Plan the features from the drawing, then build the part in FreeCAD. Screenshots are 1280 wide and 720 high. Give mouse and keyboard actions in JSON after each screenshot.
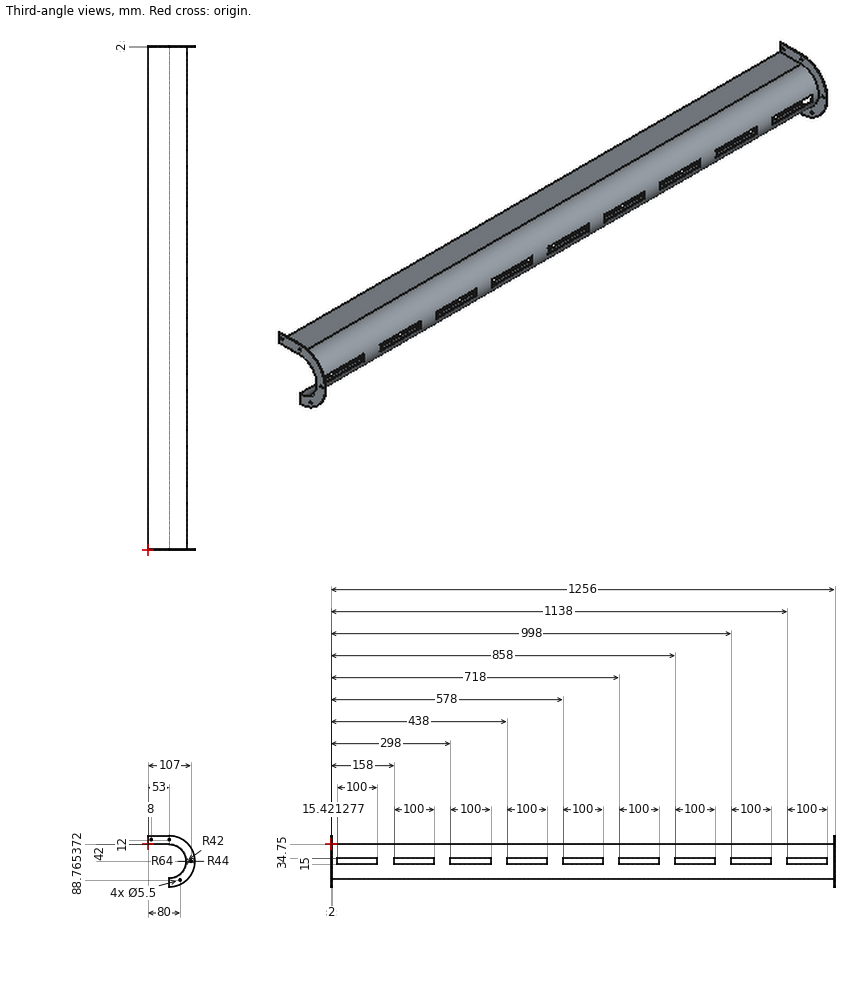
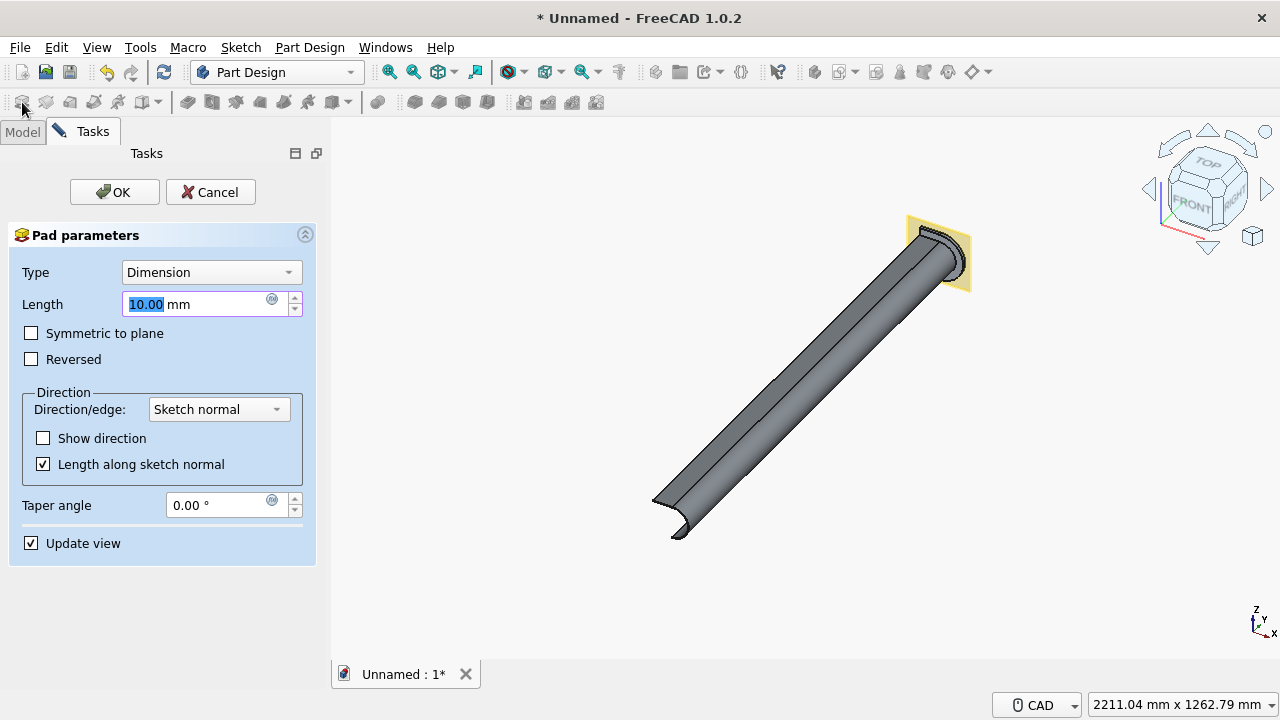
{"action": "type", "text": "2"}
{"action": "key", "text": "Tab"}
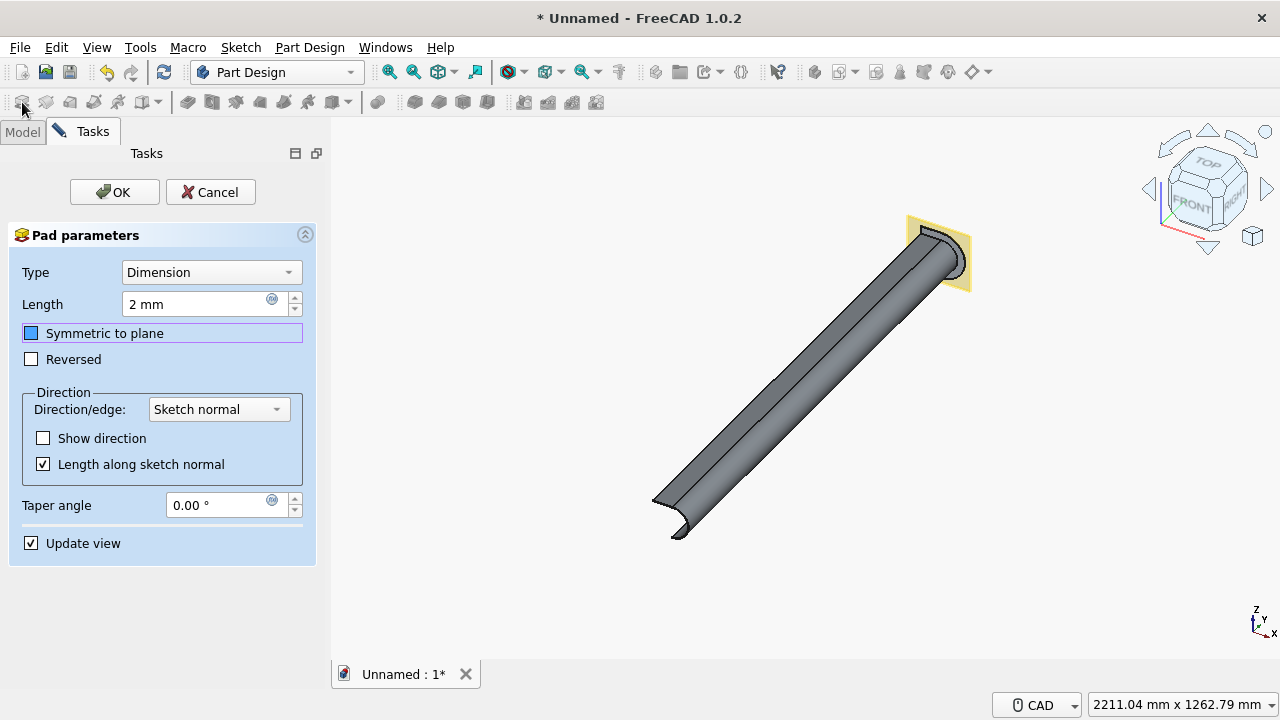
{"action": "left_click", "coordinate": [30, 359]}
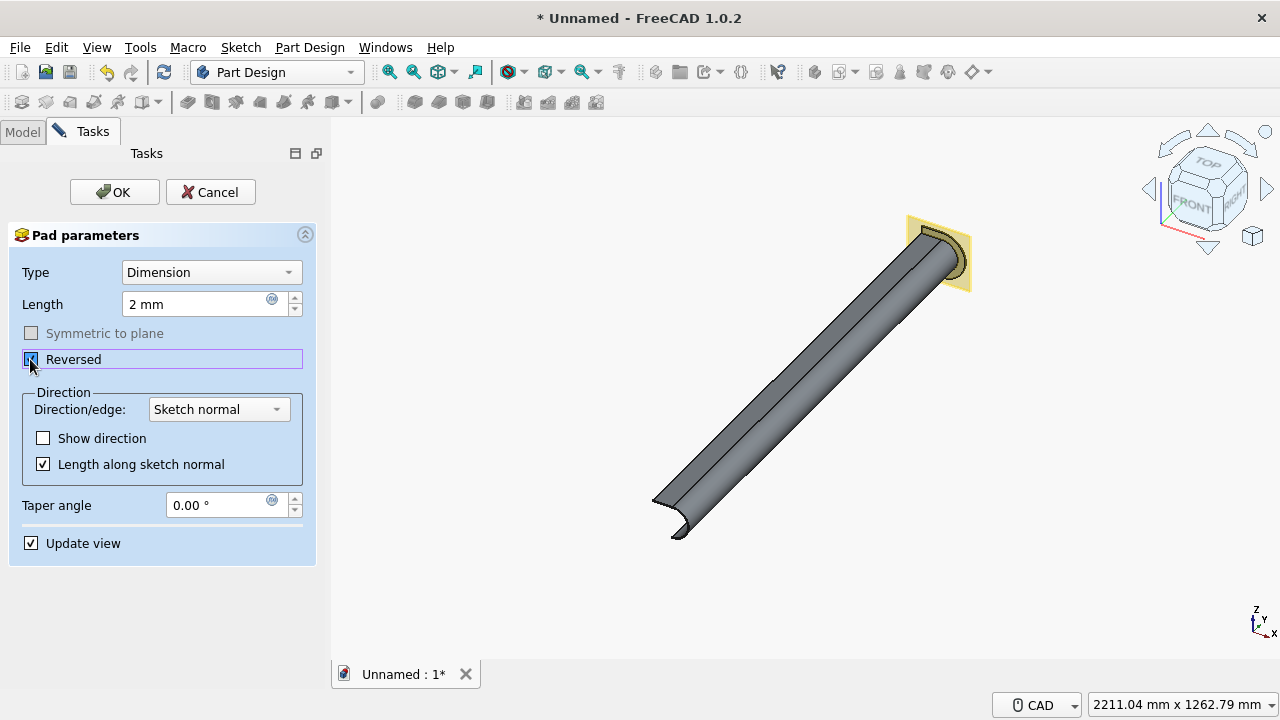
{"action": "left_click", "coordinate": [115, 192]}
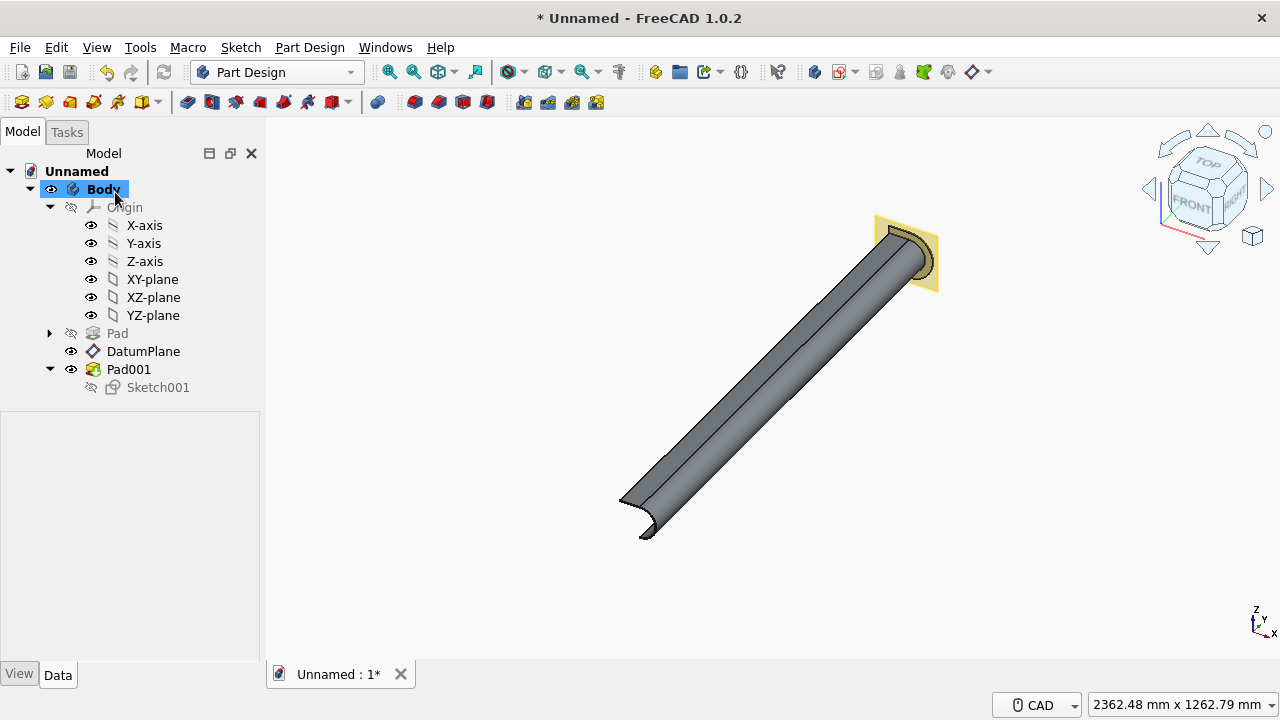
{"action": "left_click", "coordinate": [116, 351]}
{"action": "key", "text": "space"}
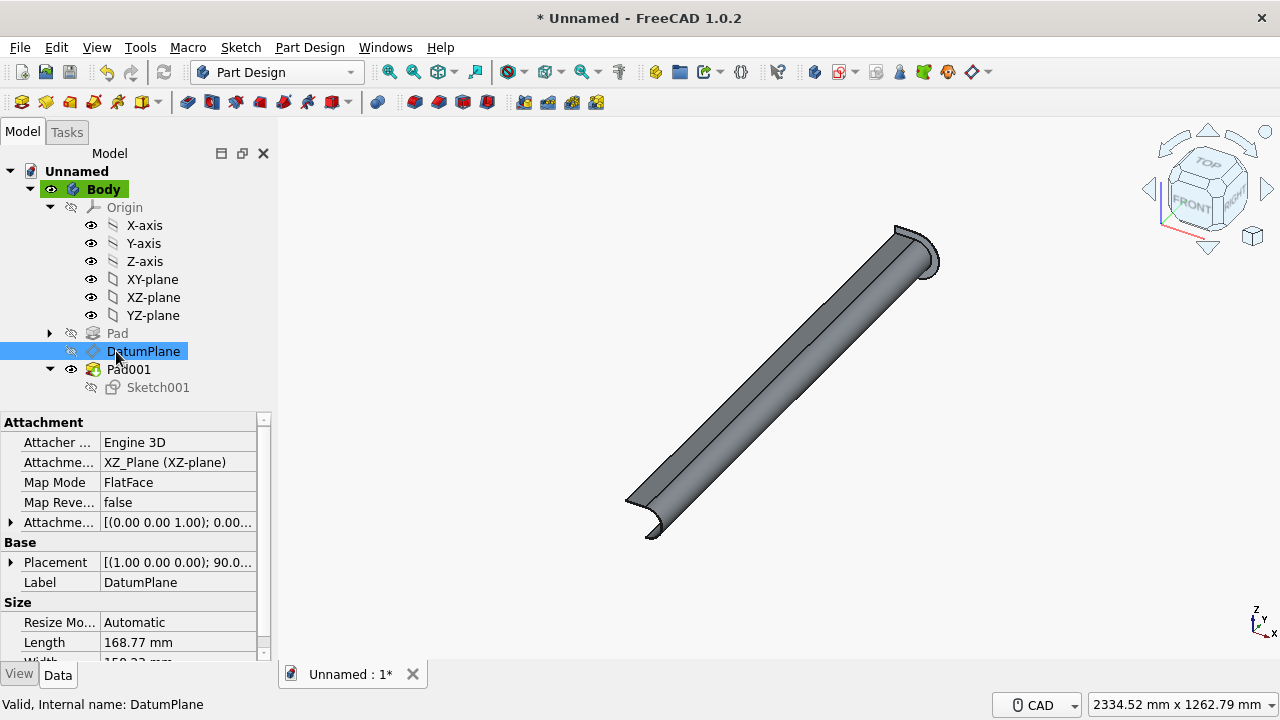
{"action": "left_click", "coordinate": [318, 619]}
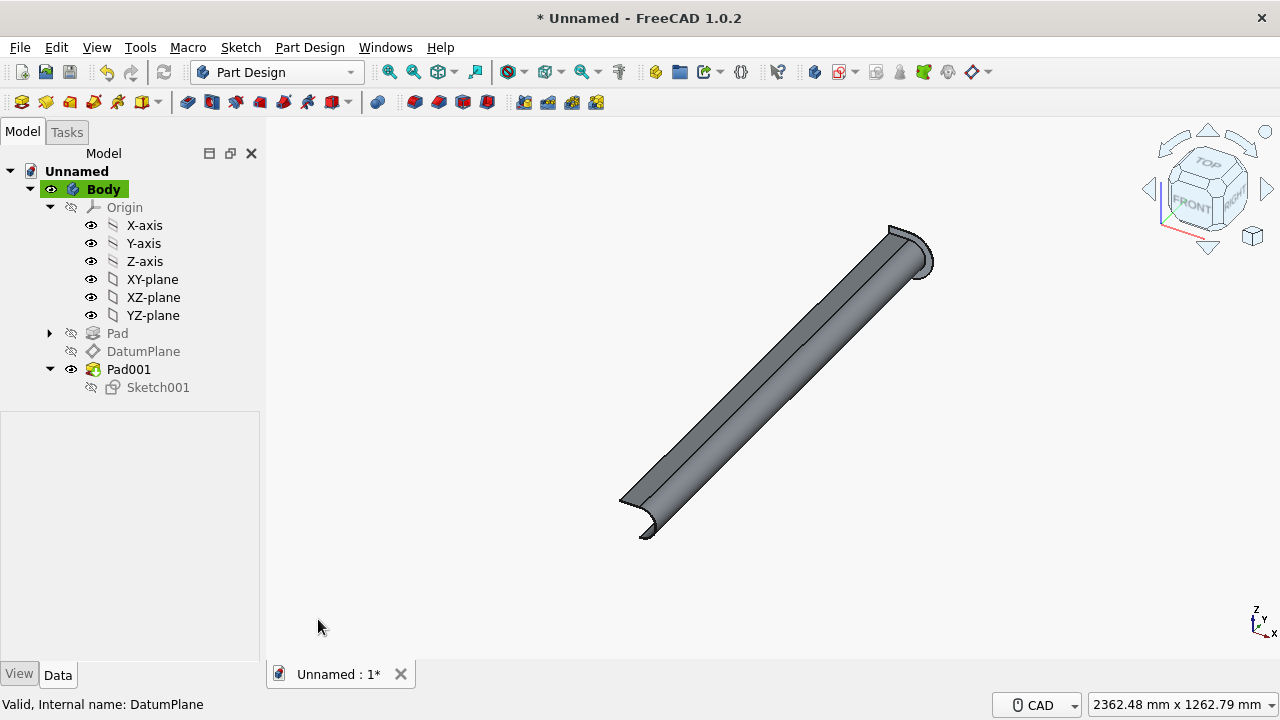
{"action": "left_click", "coordinate": [840, 72]}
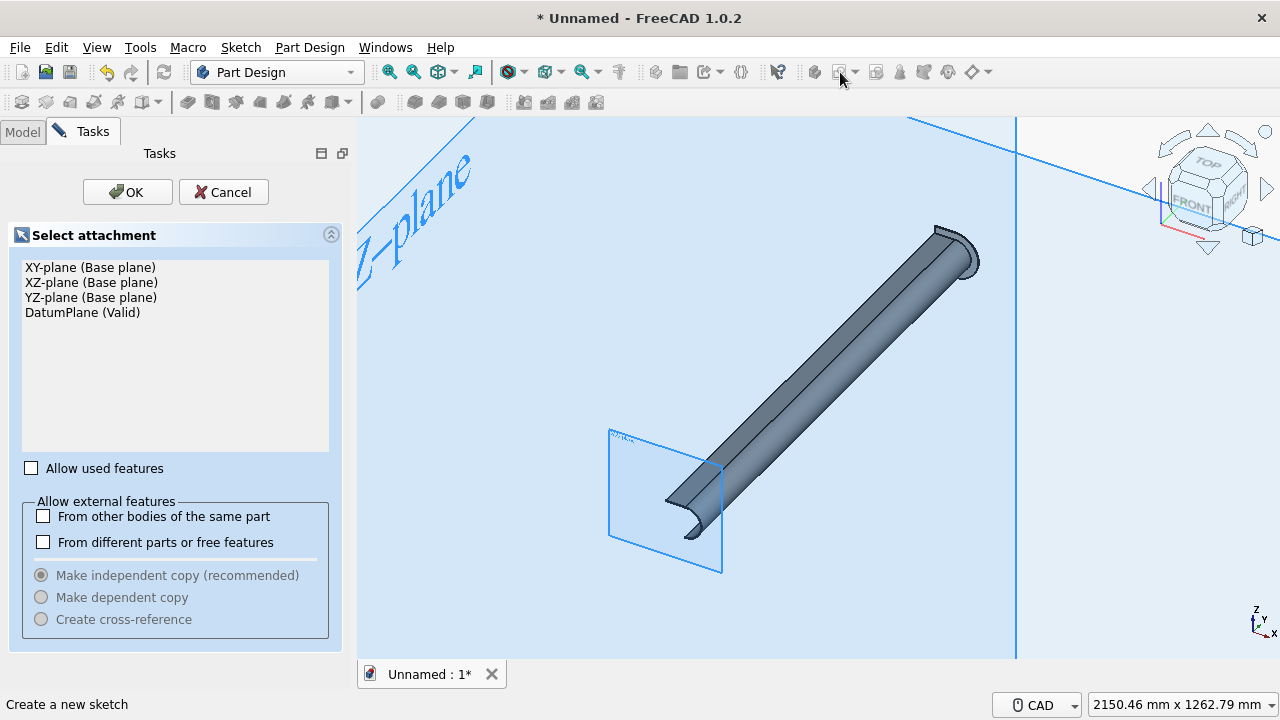
{"action": "left_click", "coordinate": [82, 282]}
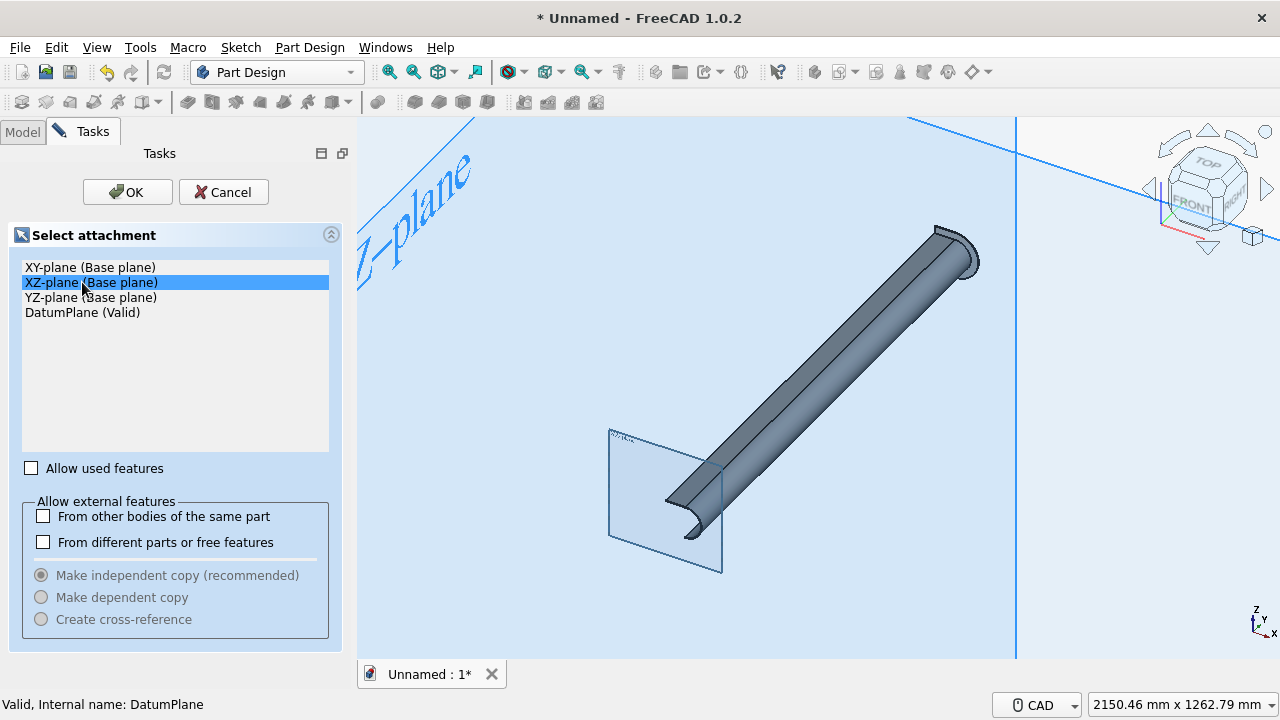
{"action": "left_click", "coordinate": [128, 192]}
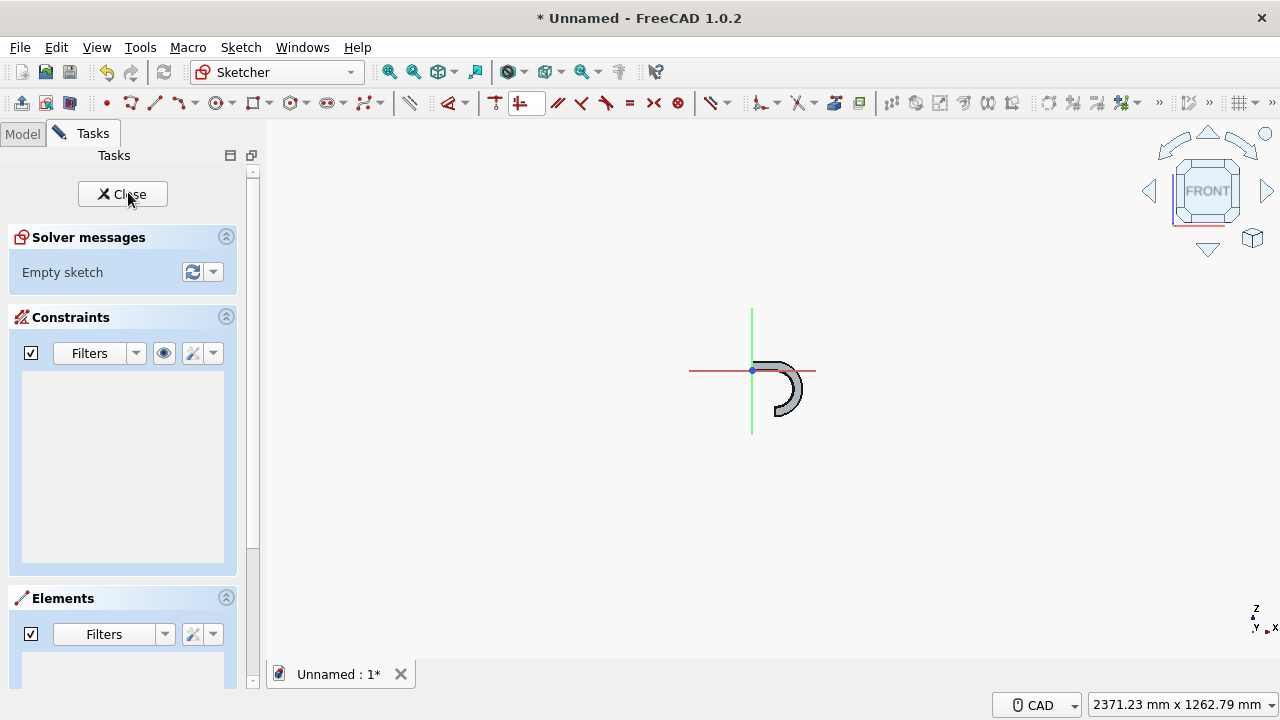
{"action": "scroll", "coordinate": [792, 389], "scroll_direction": "up", "scroll_amount": 9}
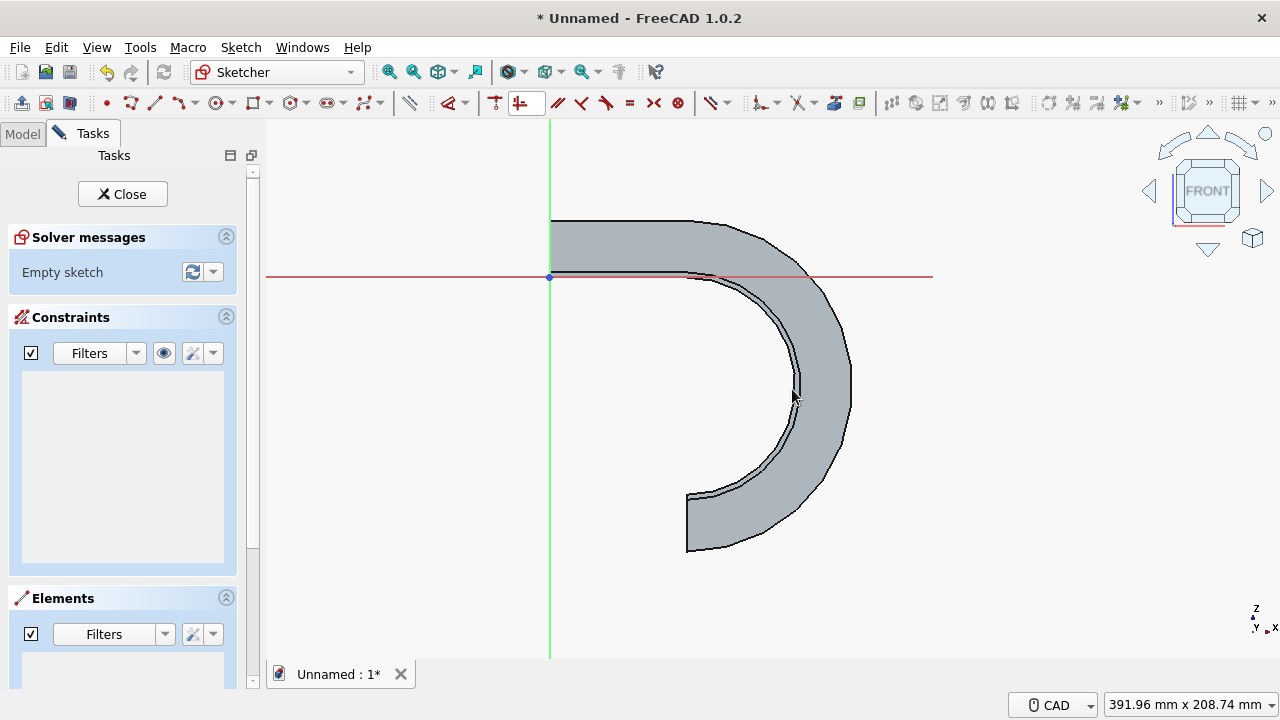
{"action": "left_click", "coordinate": [156, 104]}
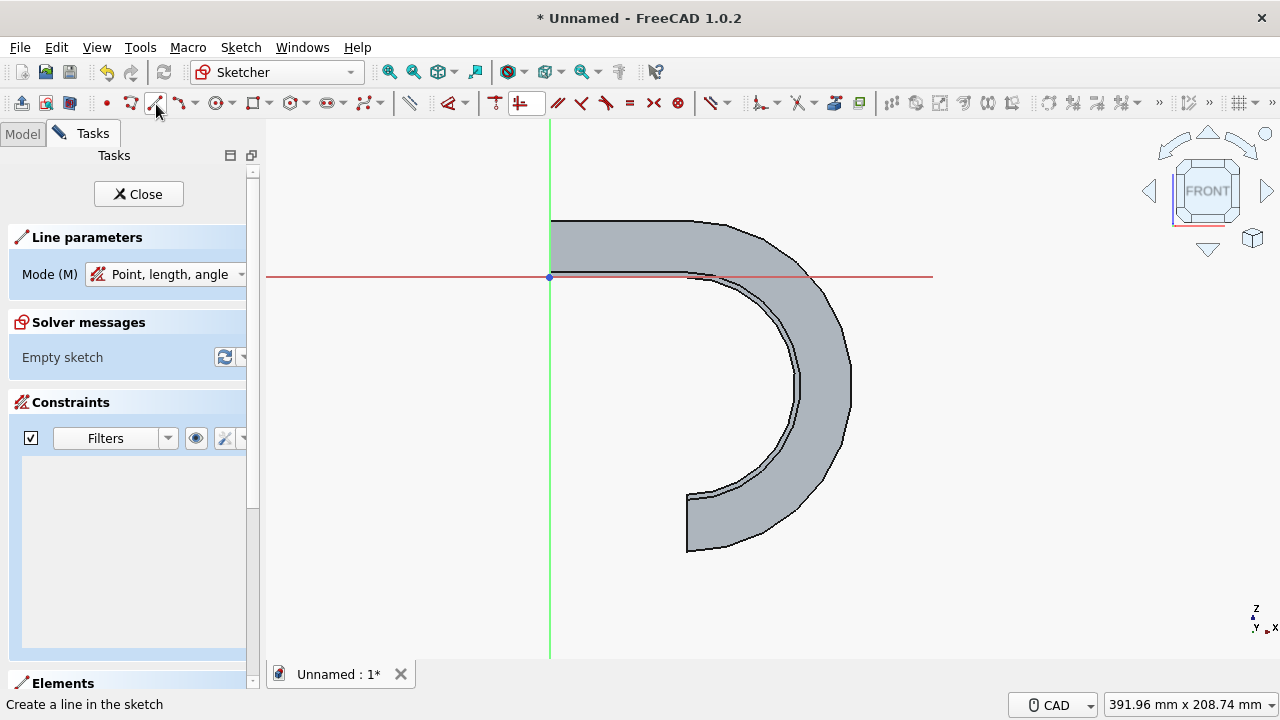
{"action": "left_click", "coordinate": [687, 495]}
{"action": "left_click", "coordinate": [687, 552]}